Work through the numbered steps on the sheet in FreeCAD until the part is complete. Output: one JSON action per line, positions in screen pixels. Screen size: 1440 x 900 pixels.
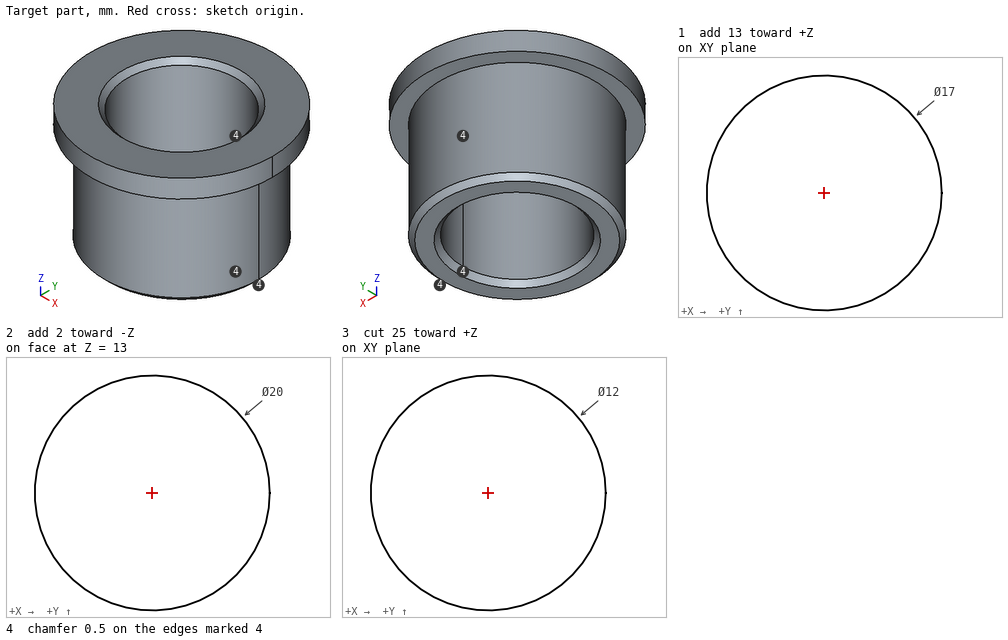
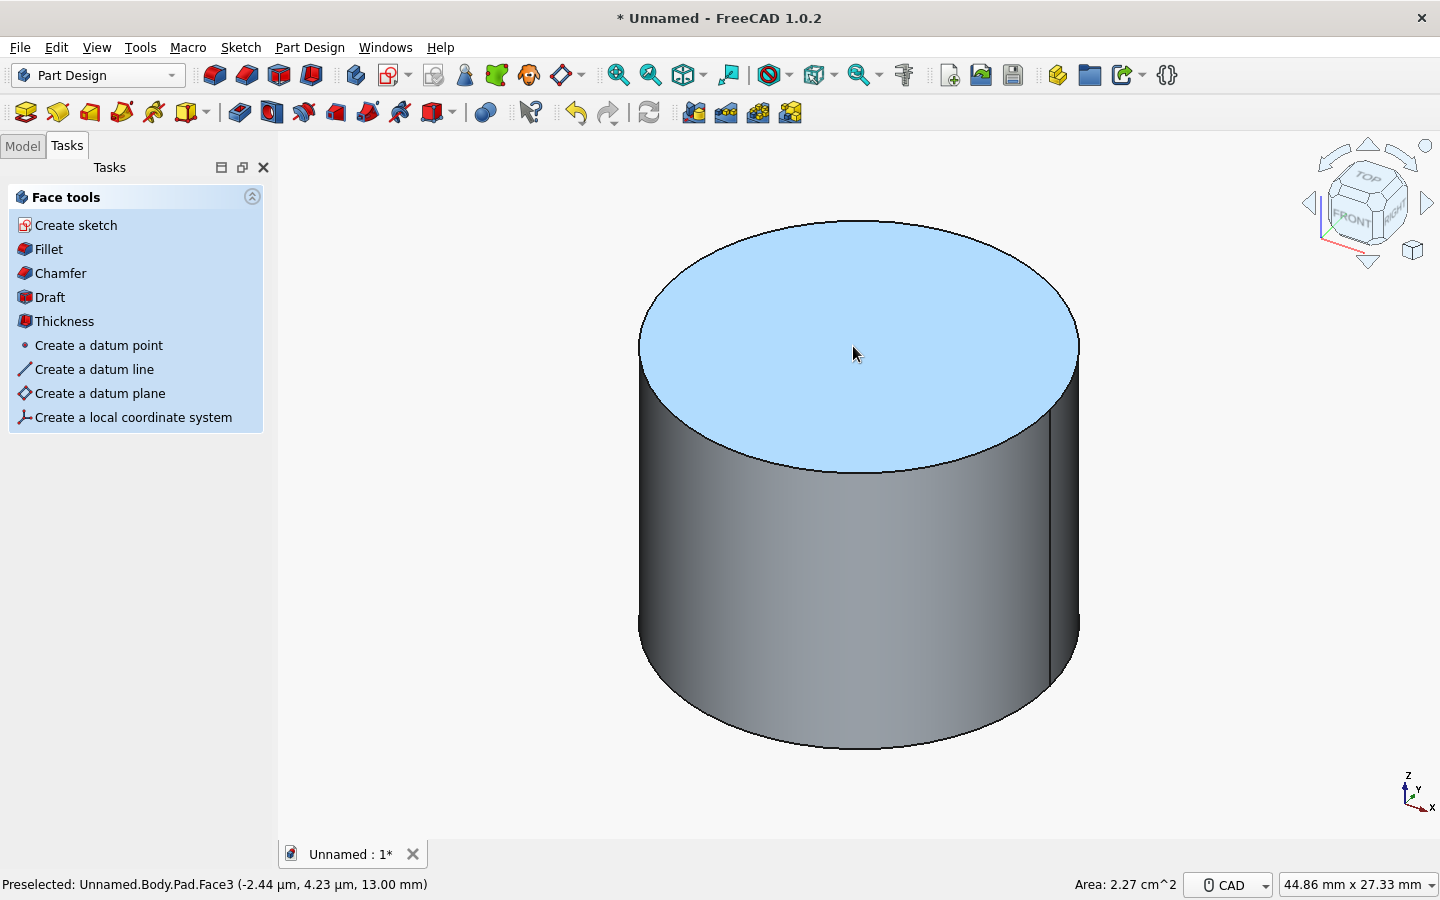
{"action": "left_click", "coordinate": [388, 76]}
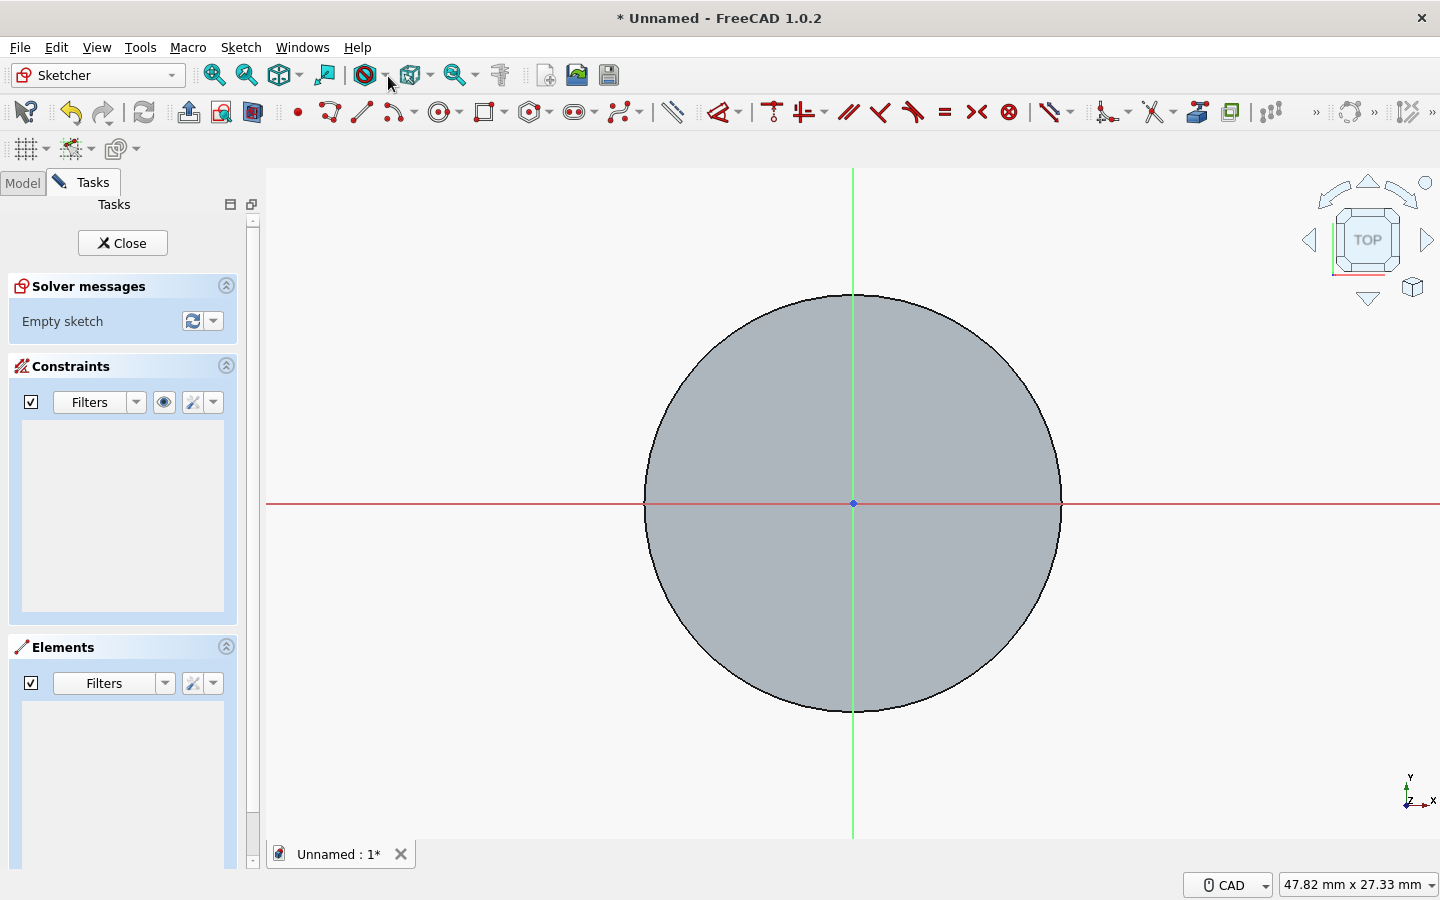
{"action": "key", "text": "g c"}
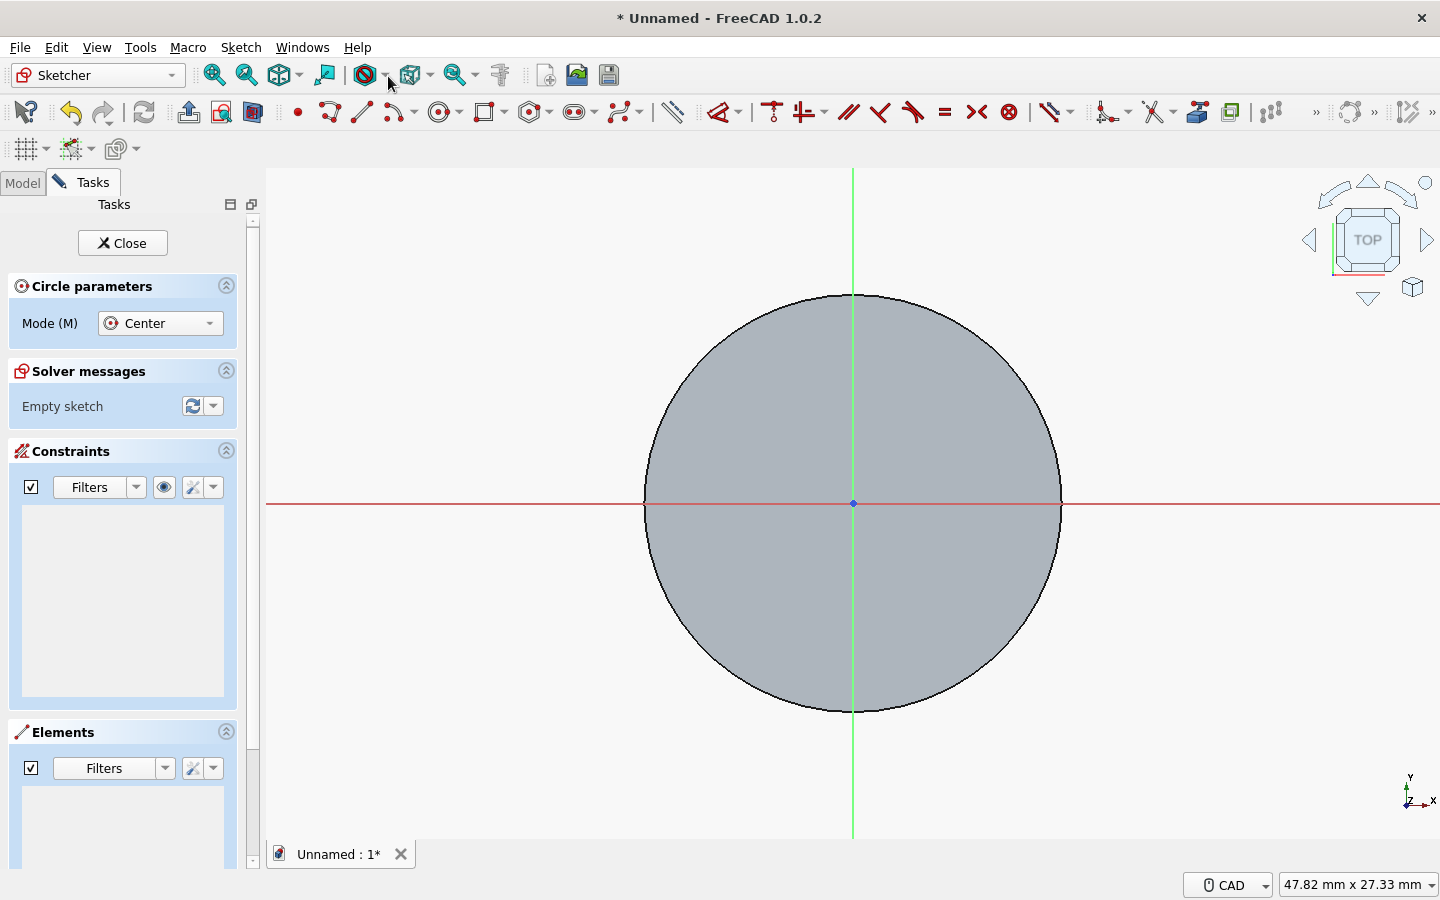
{"action": "left_click", "coordinate": [853, 504]}
{"action": "left_click", "coordinate": [1027, 330]}
{"action": "key", "text": "Escape"}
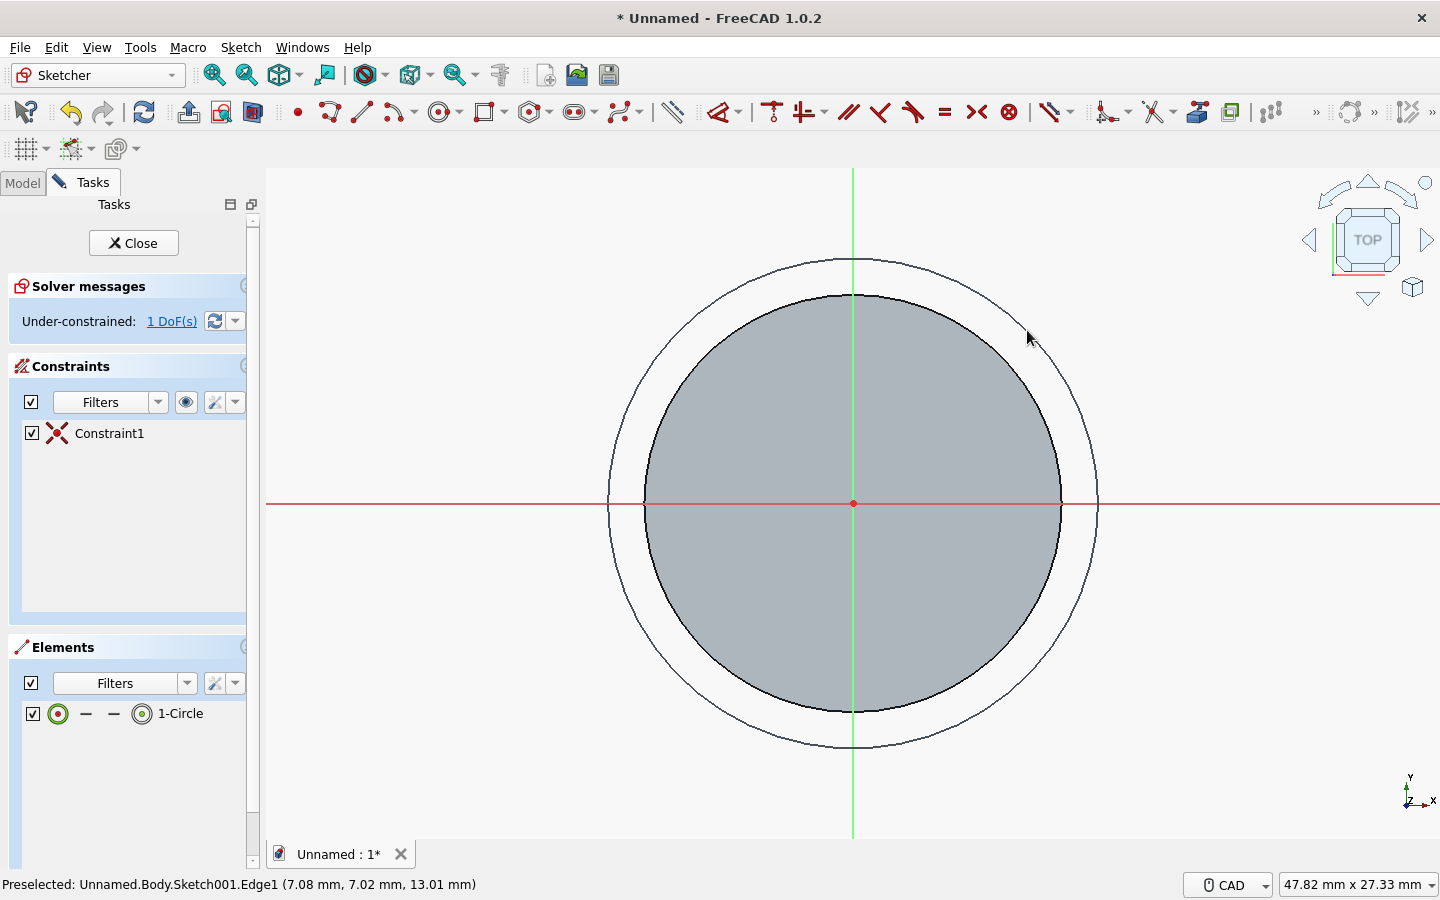
{"action": "left_click", "coordinate": [1026, 330]}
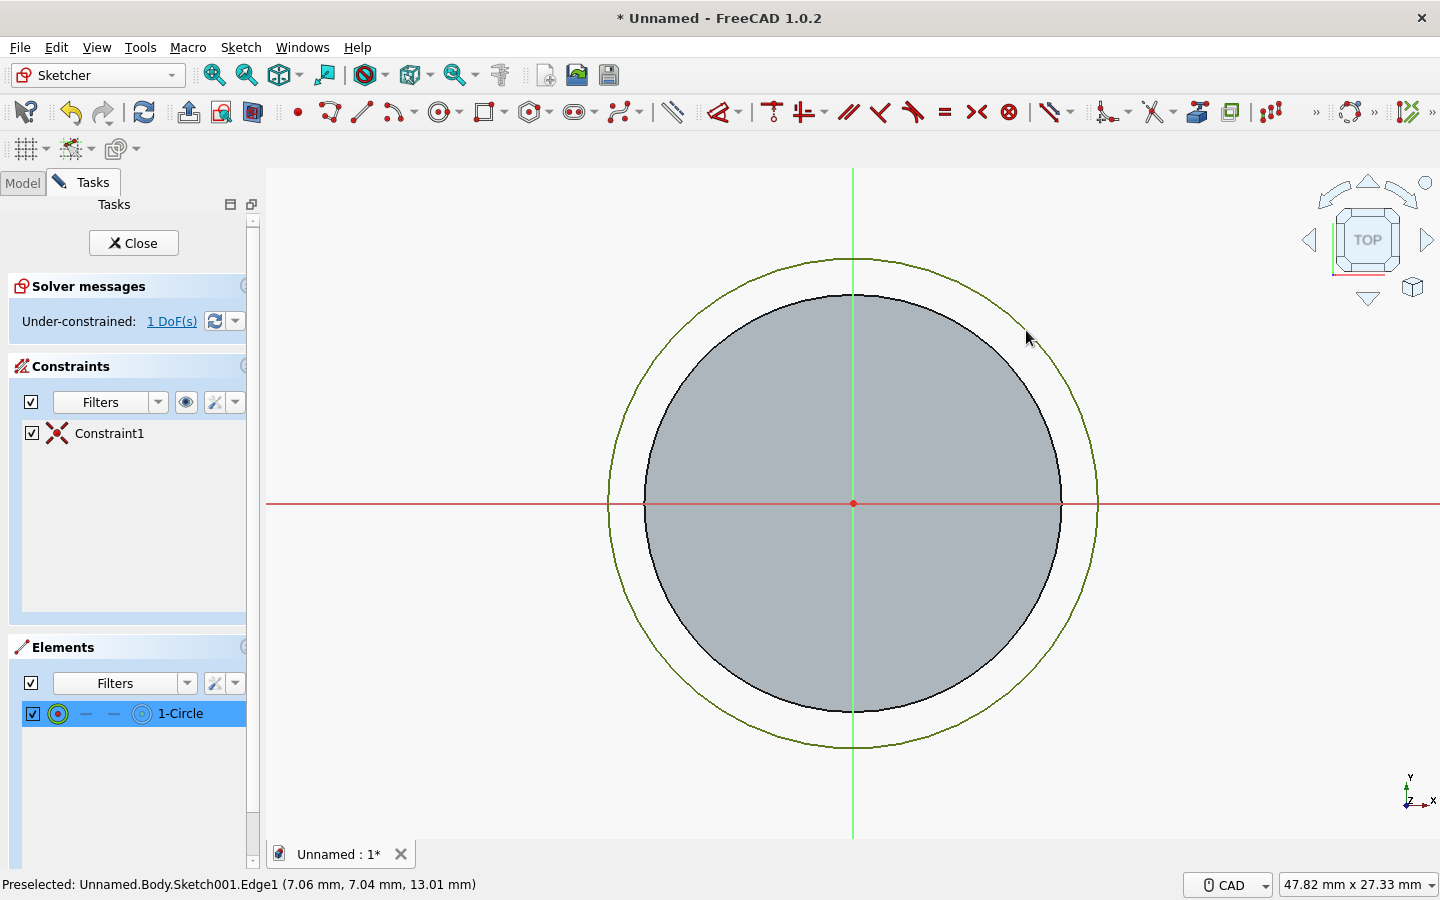
{"action": "left_click", "coordinate": [740, 112]}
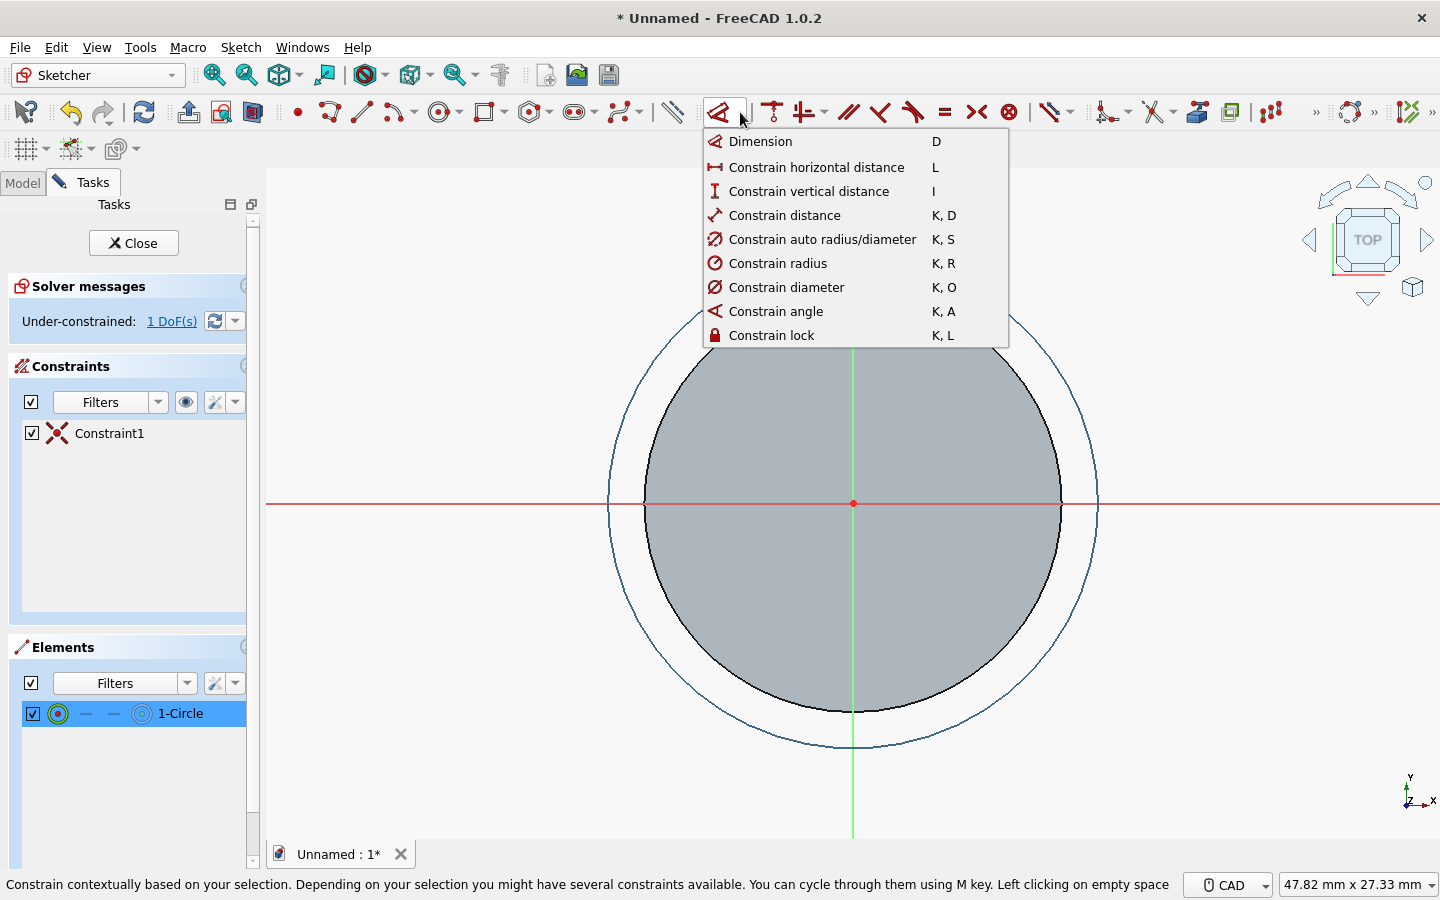
{"action": "left_click", "coordinate": [856, 287]}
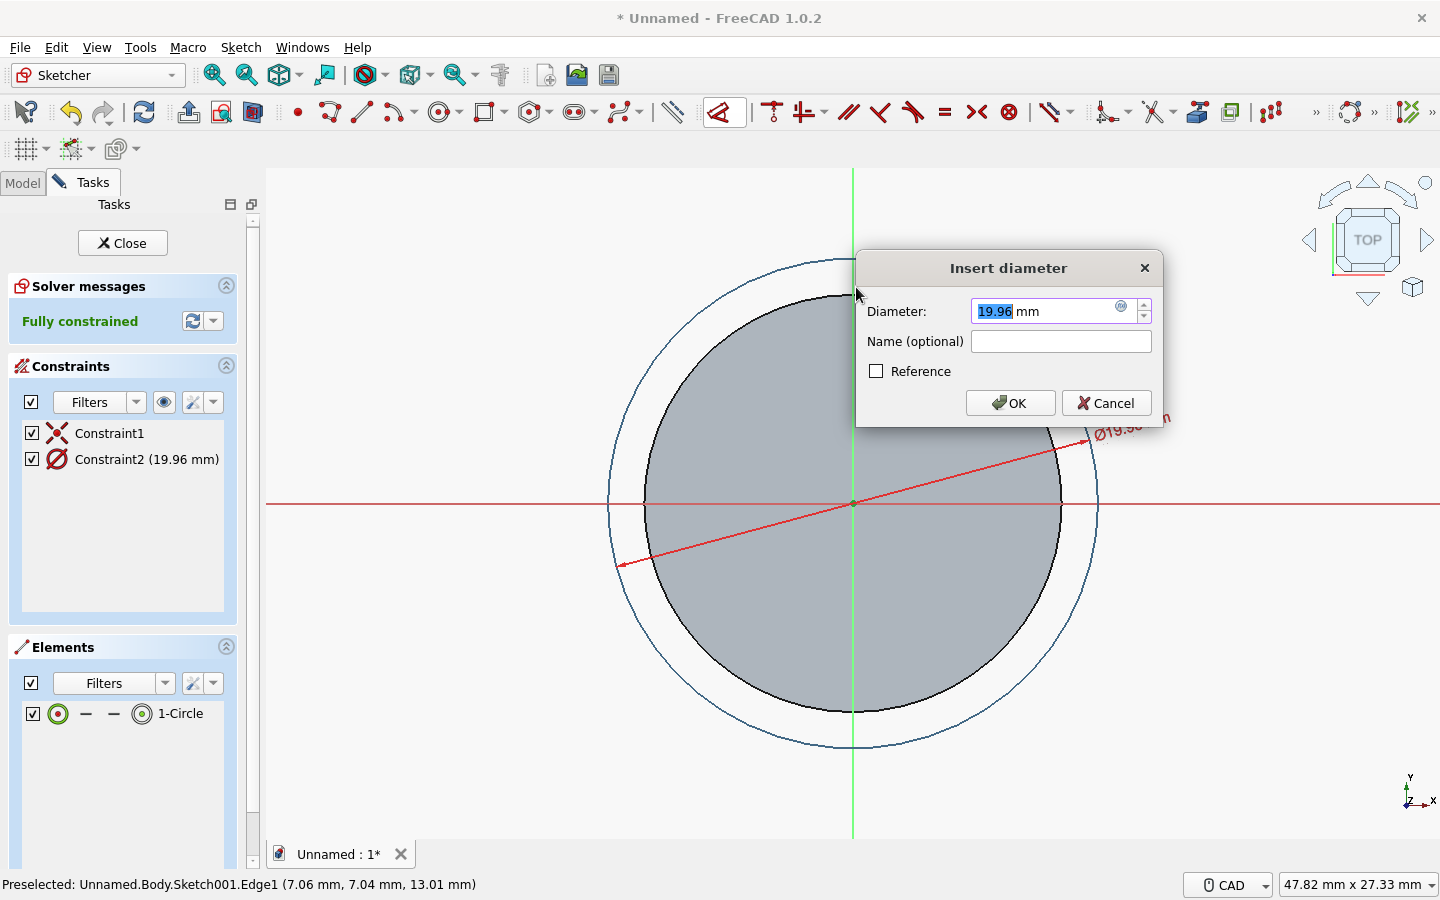
{"action": "type", "text": "20"}
{"action": "key", "text": "Return"}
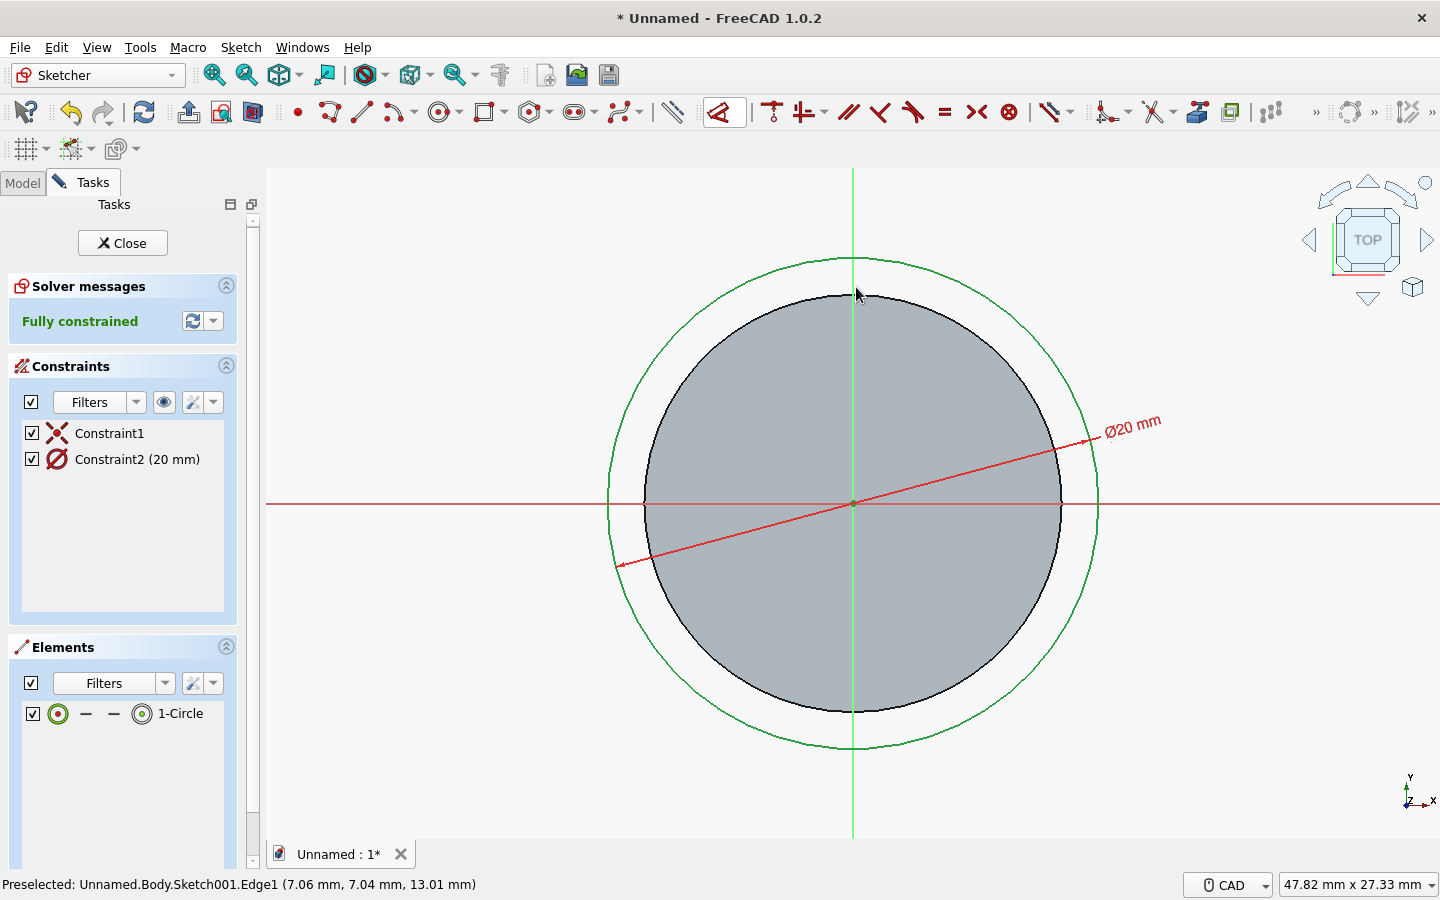
{"action": "left_click", "coordinate": [123, 243]}